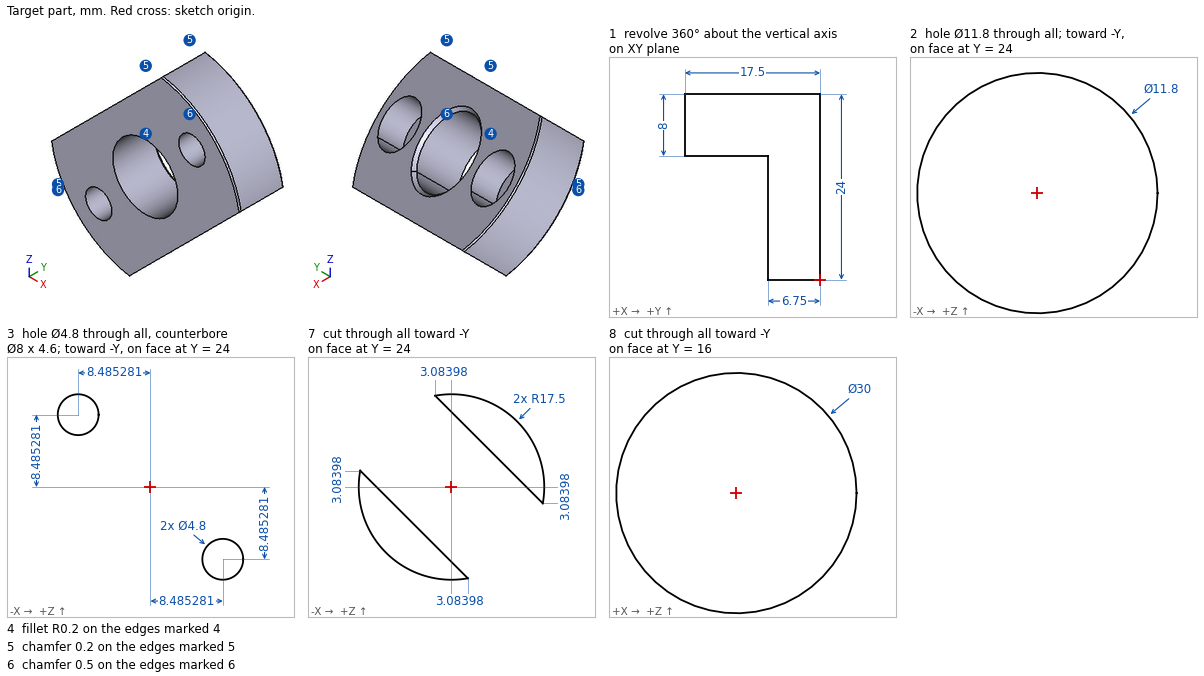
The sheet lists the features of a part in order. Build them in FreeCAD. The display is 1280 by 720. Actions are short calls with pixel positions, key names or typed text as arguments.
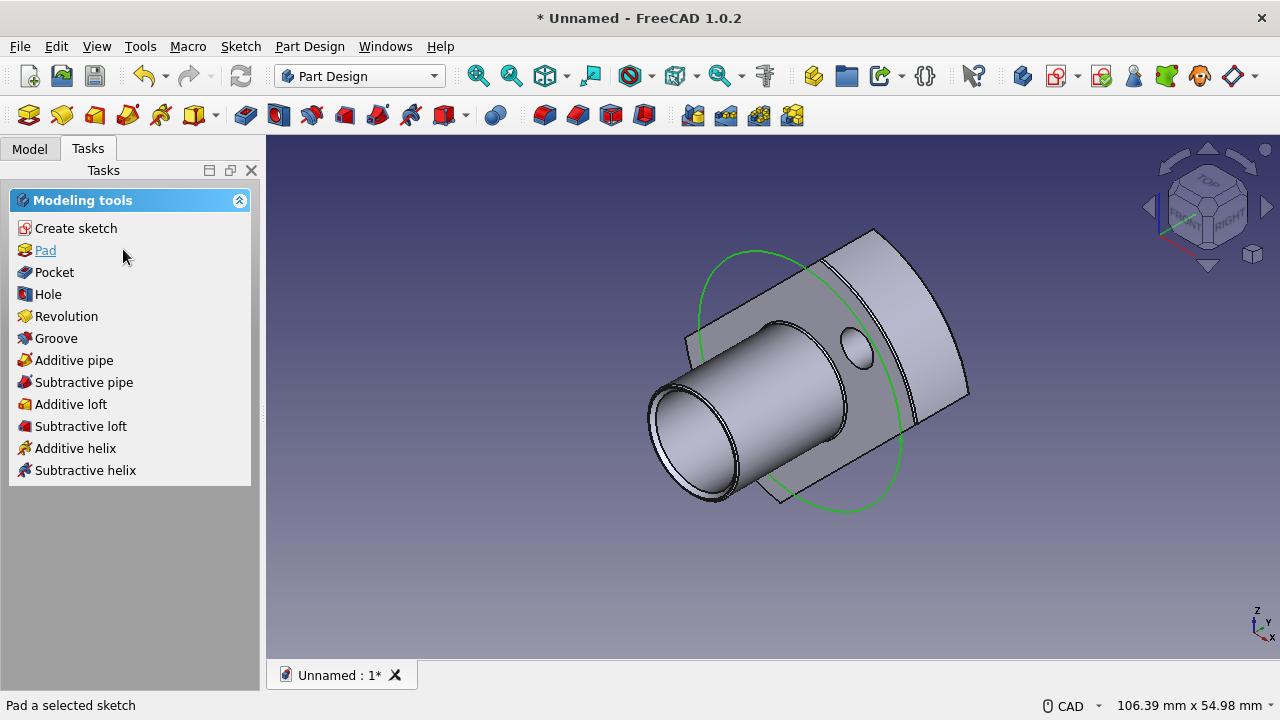
click(246, 116)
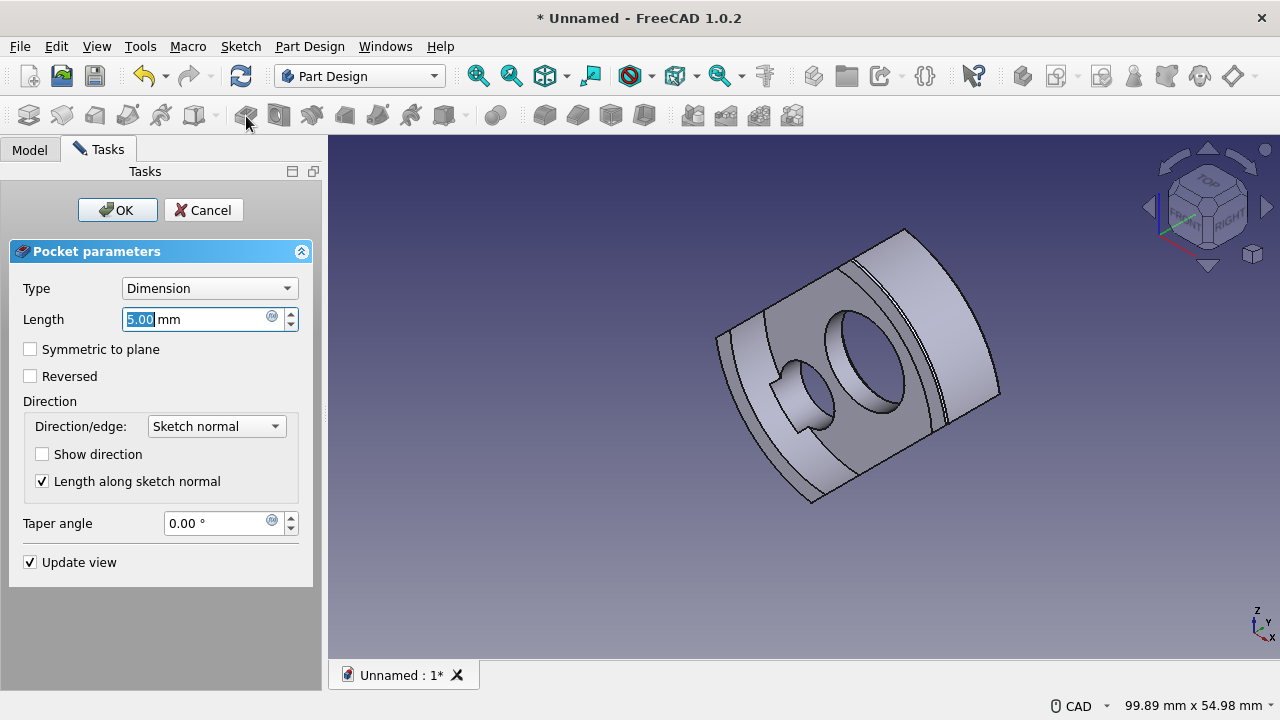
click(210, 288)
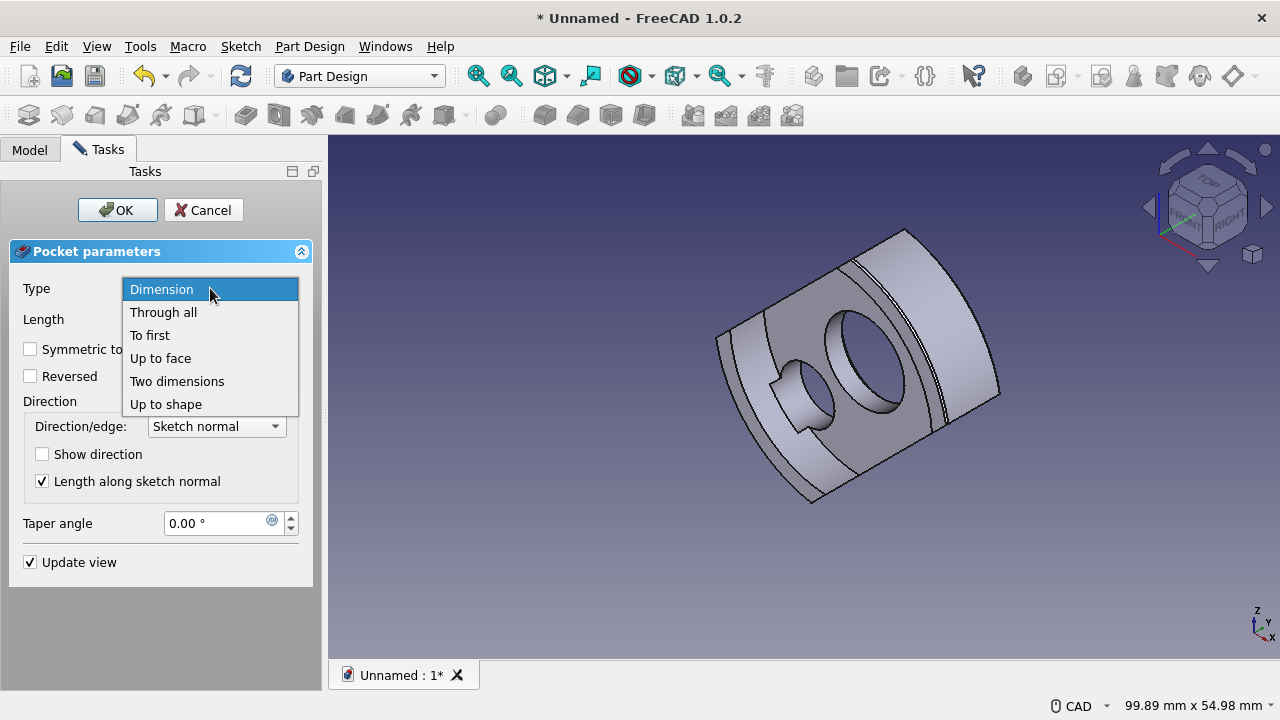
click(208, 312)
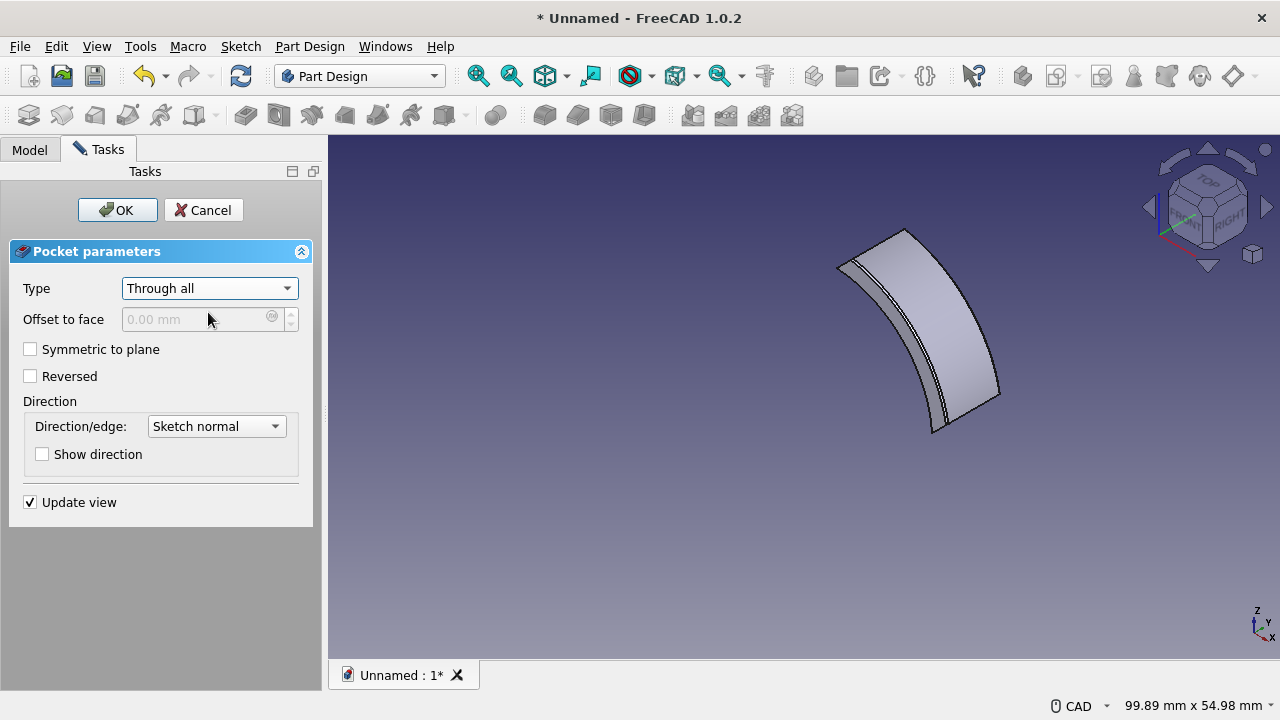
click(31, 376)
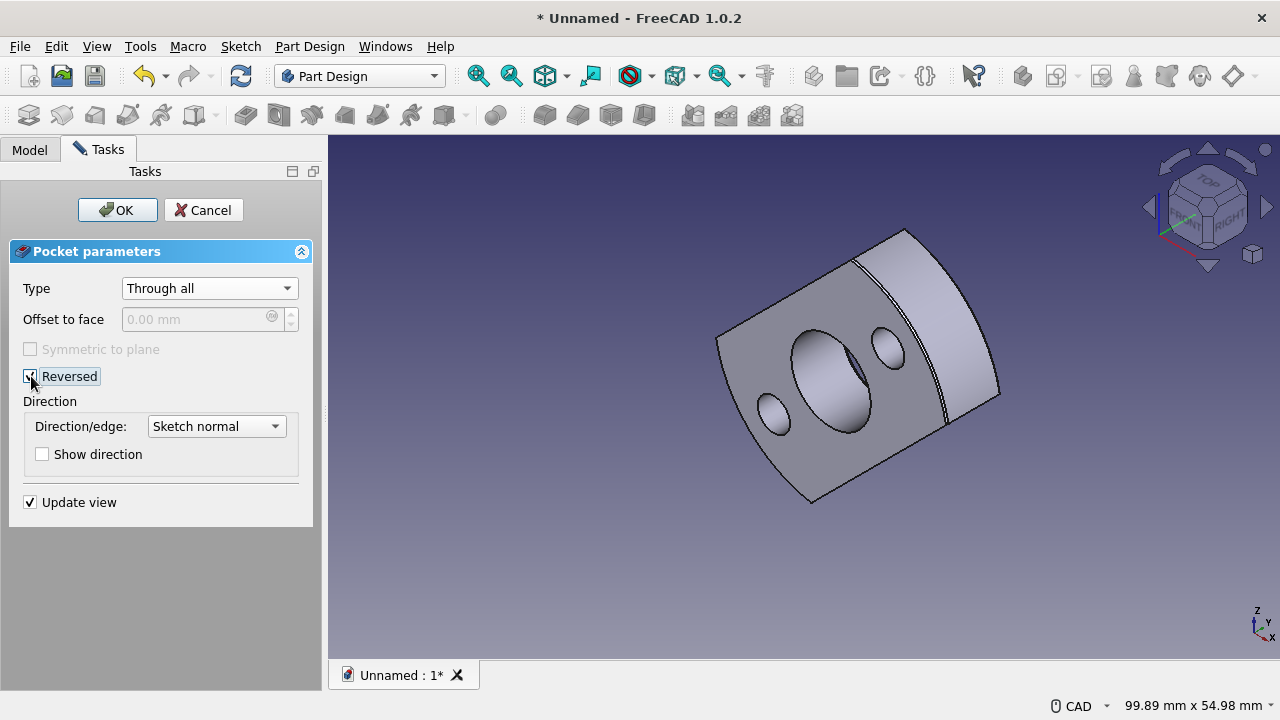
click(118, 210)